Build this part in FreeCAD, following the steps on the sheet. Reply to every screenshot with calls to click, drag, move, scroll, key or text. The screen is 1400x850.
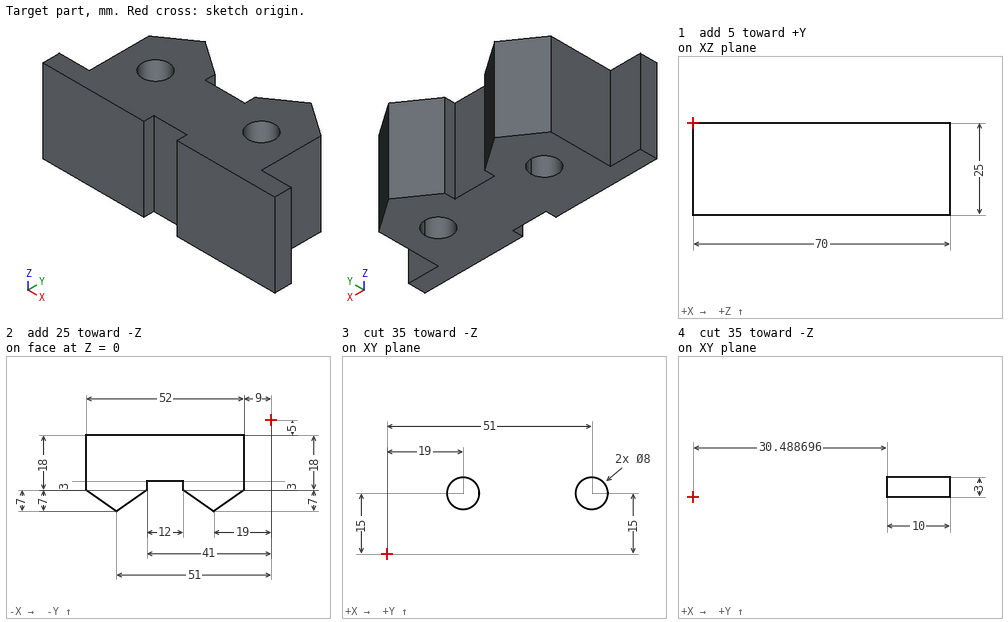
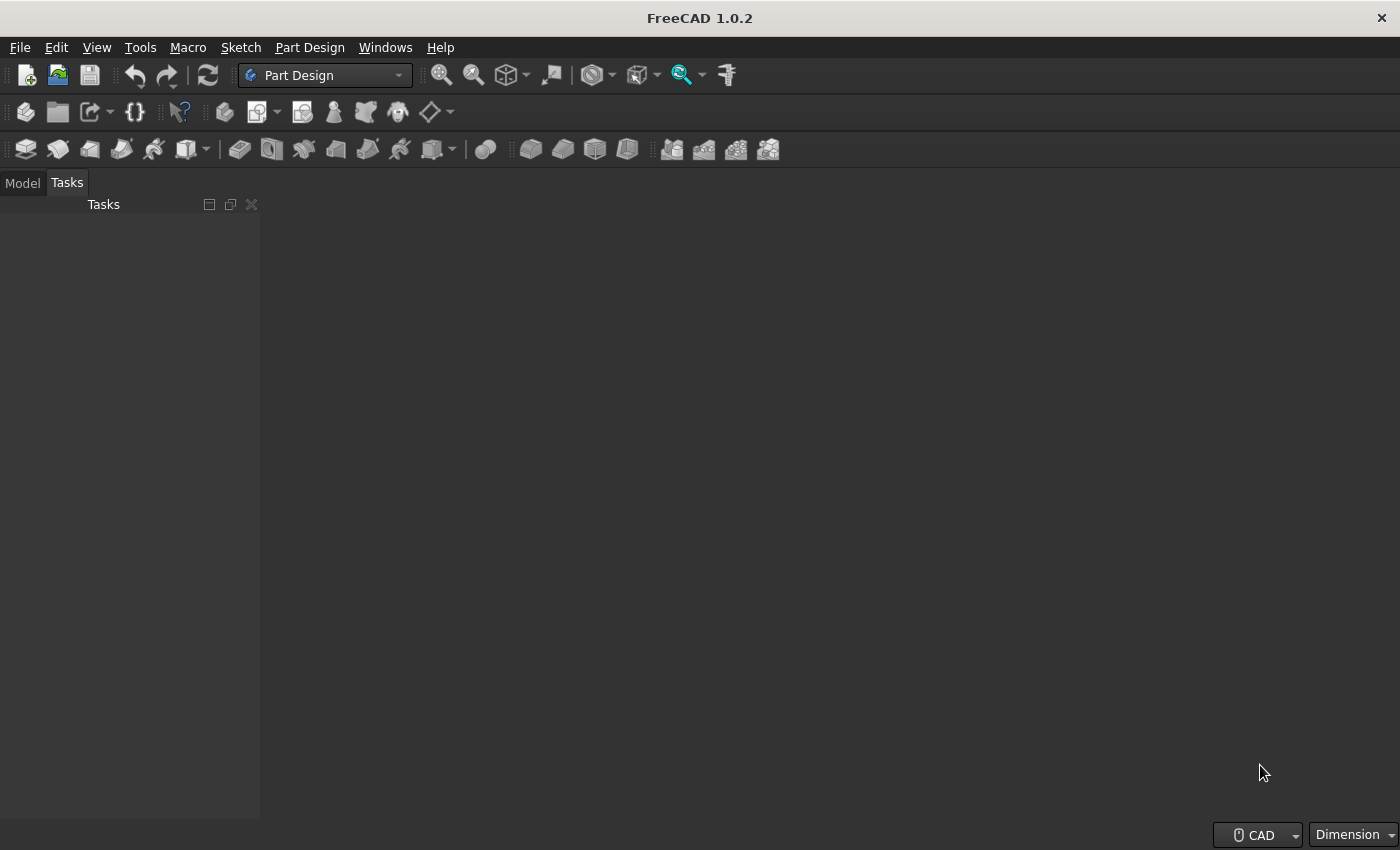
key(ctrl+n)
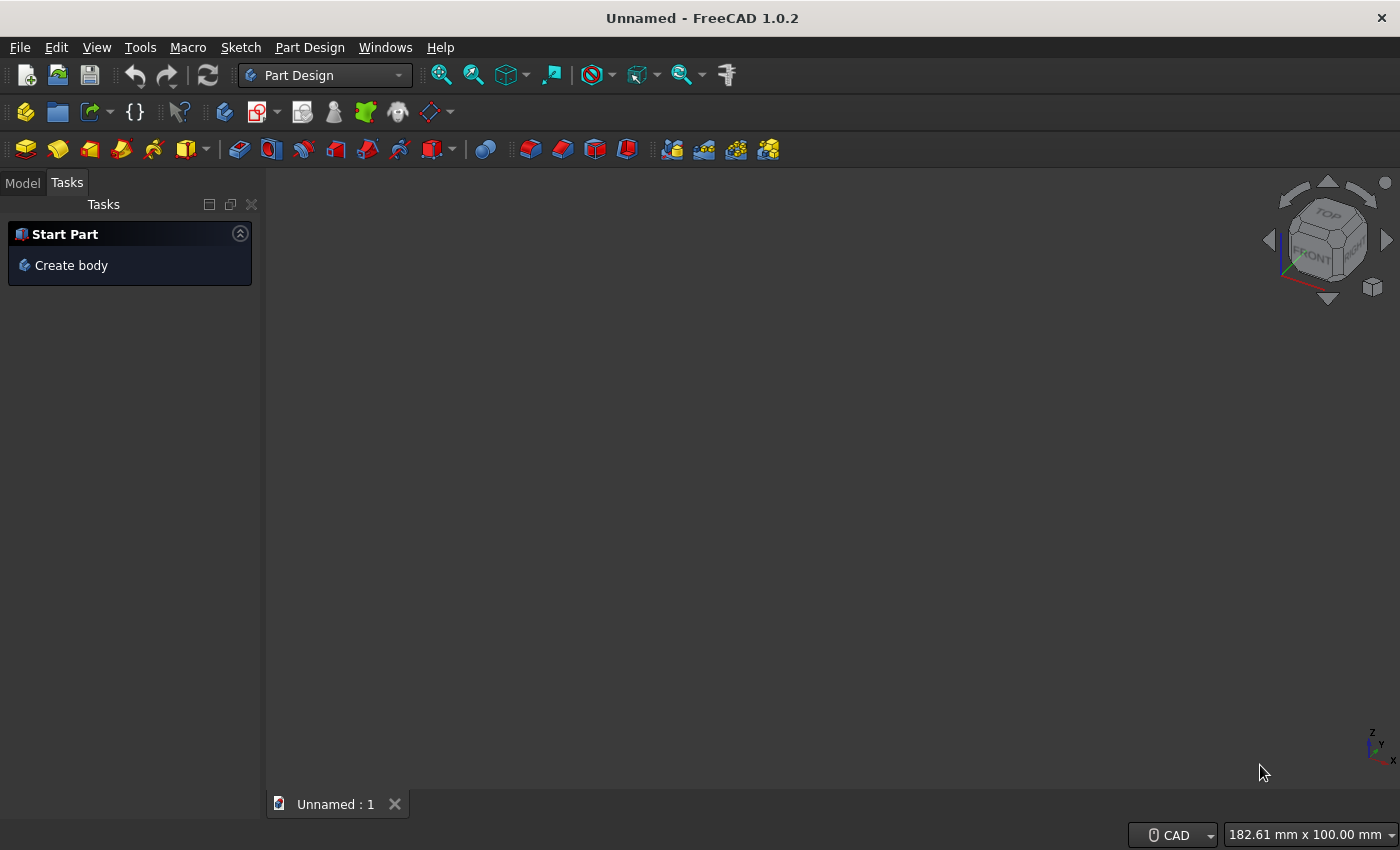
click(258, 112)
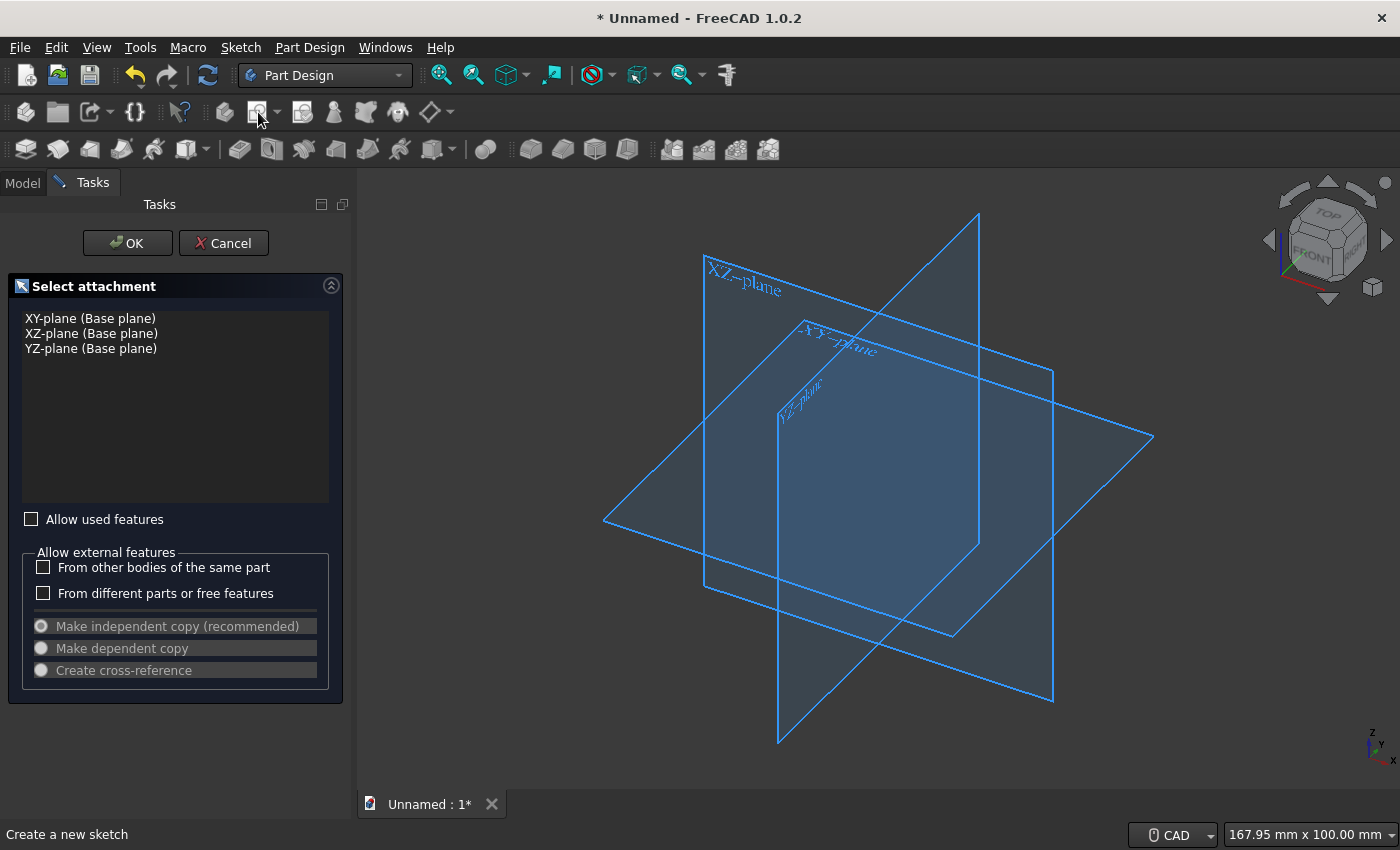
click(82, 334)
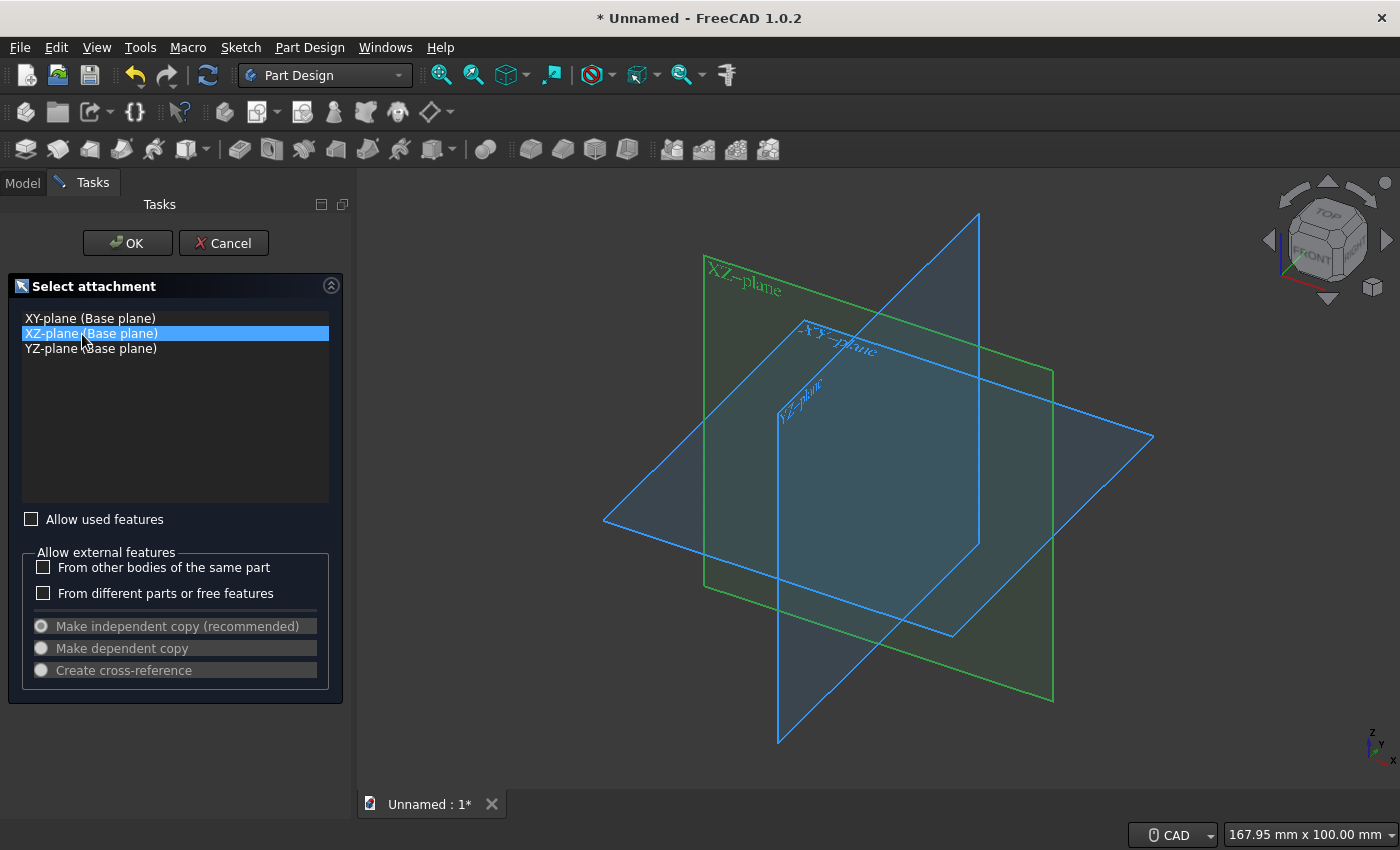
click(128, 243)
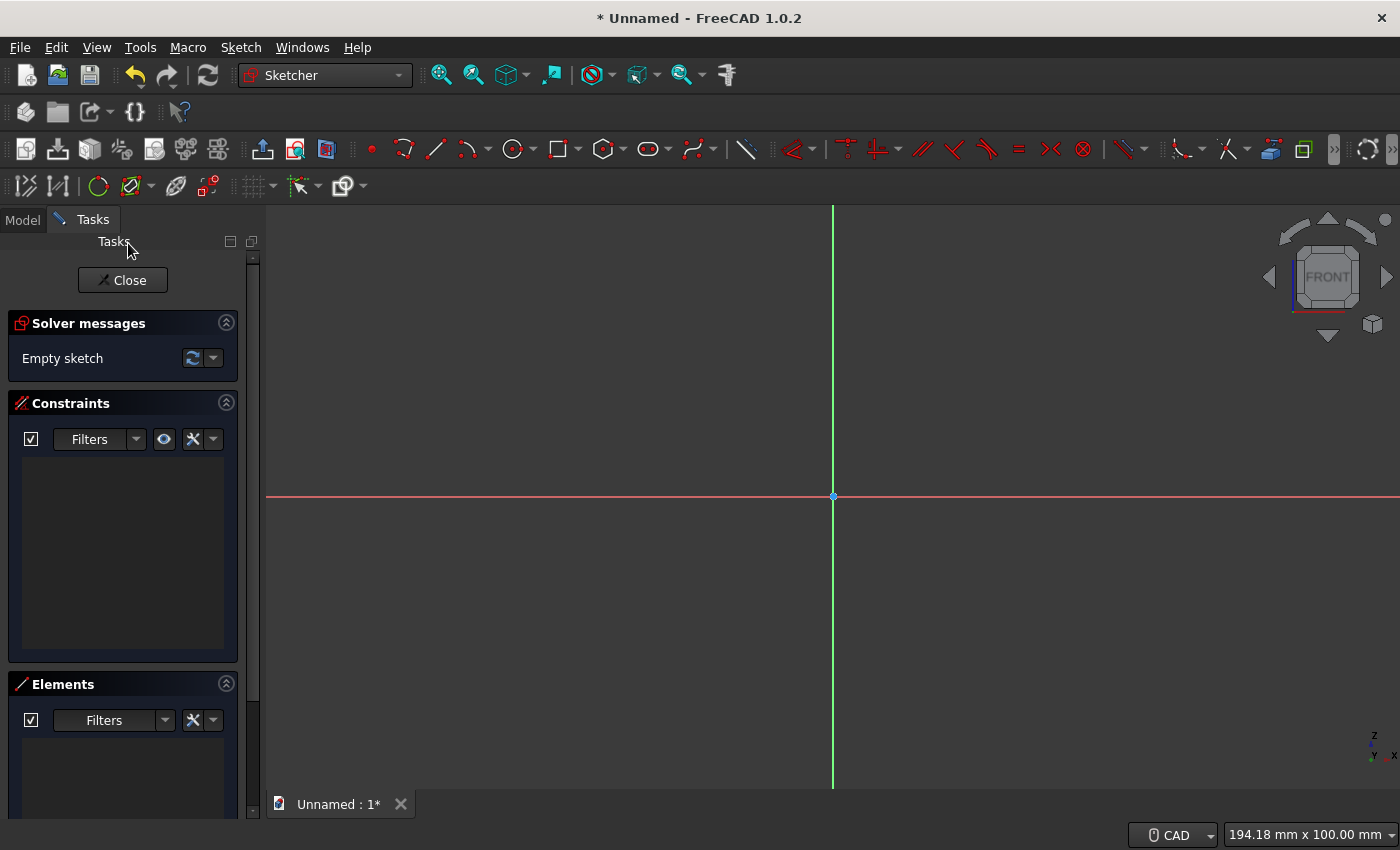
scroll(294, 233, down, 1)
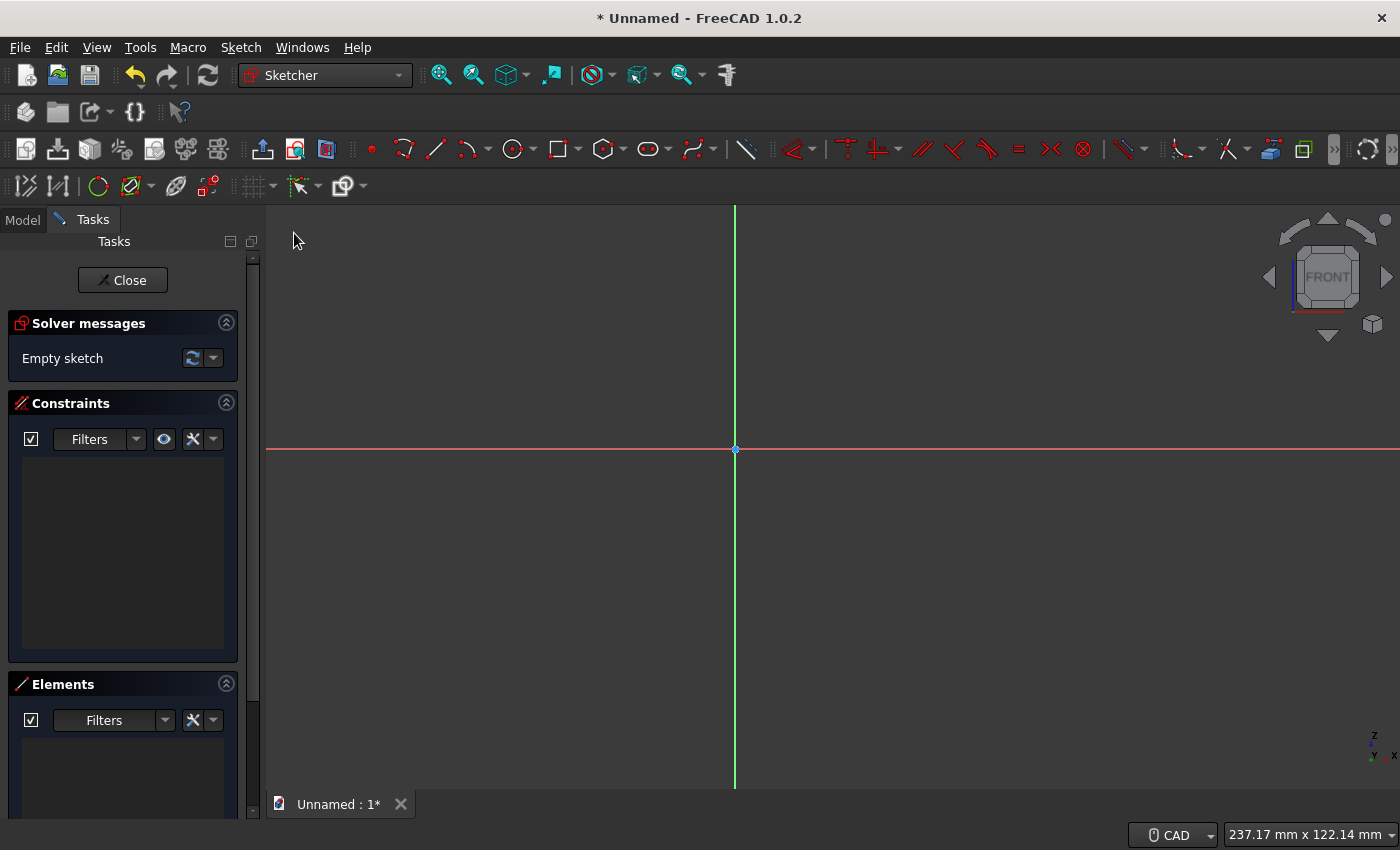
scroll(1071, 523, up, 3)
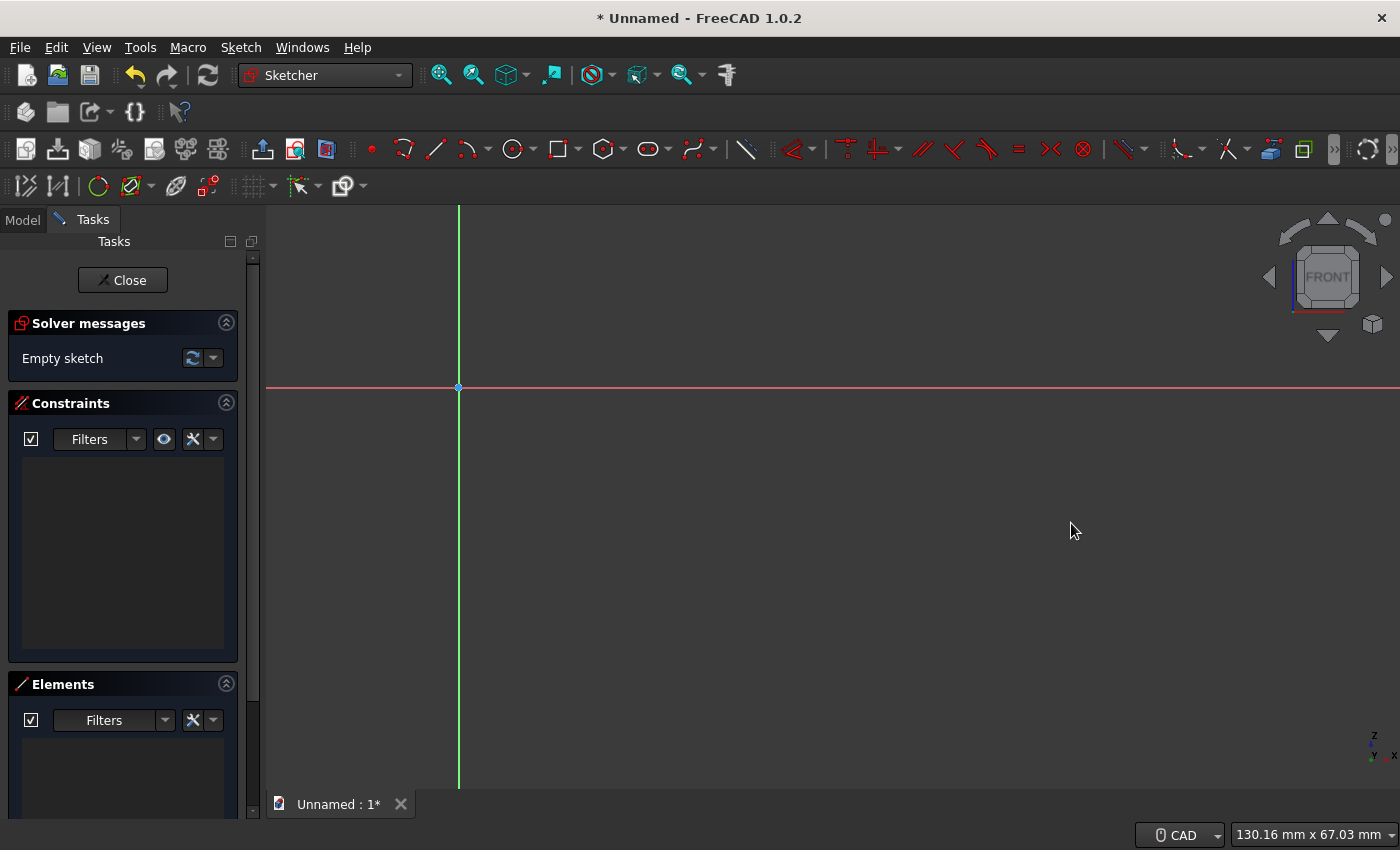
key(g)
key(r)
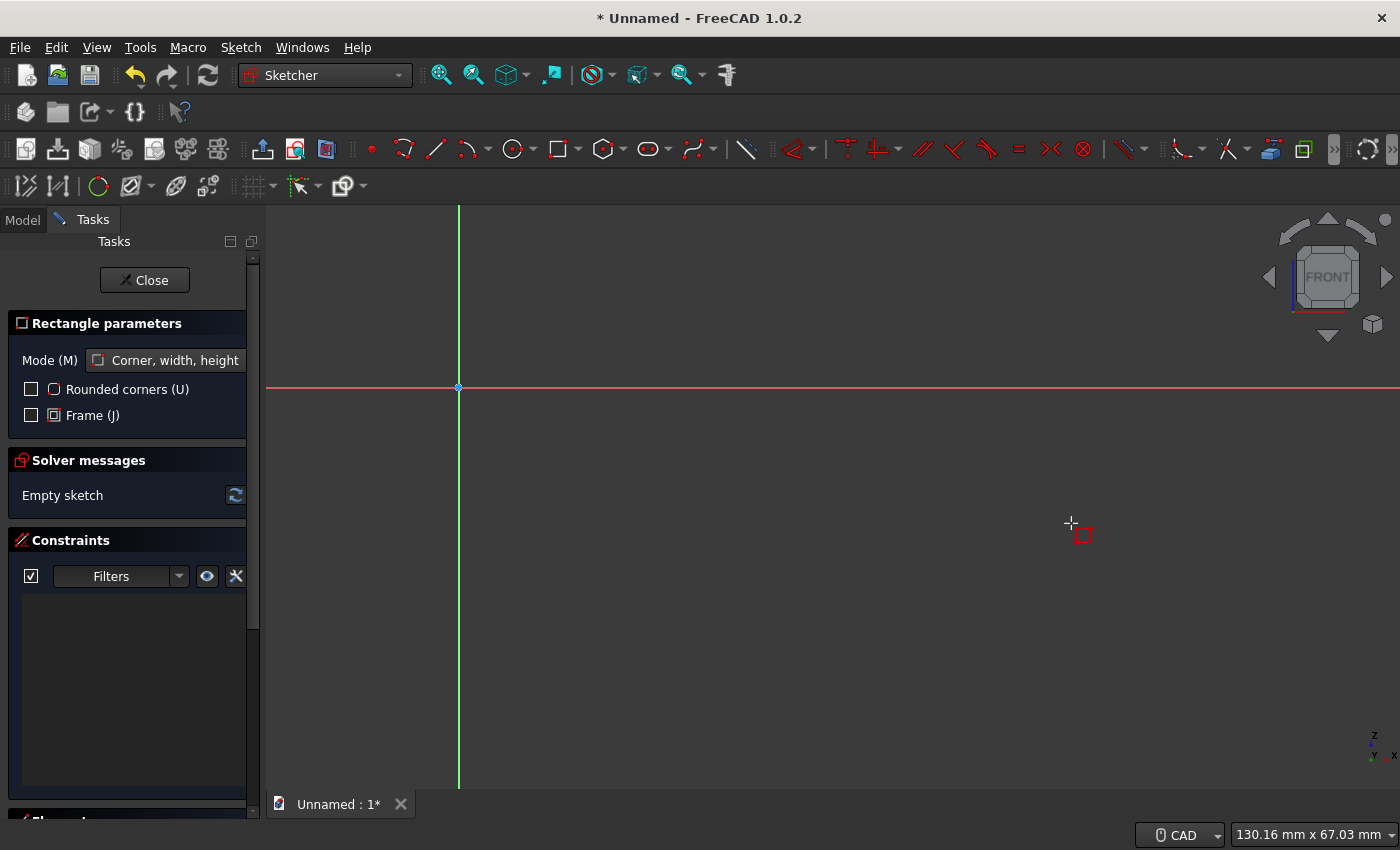
click(459, 388)
move(1069, 606)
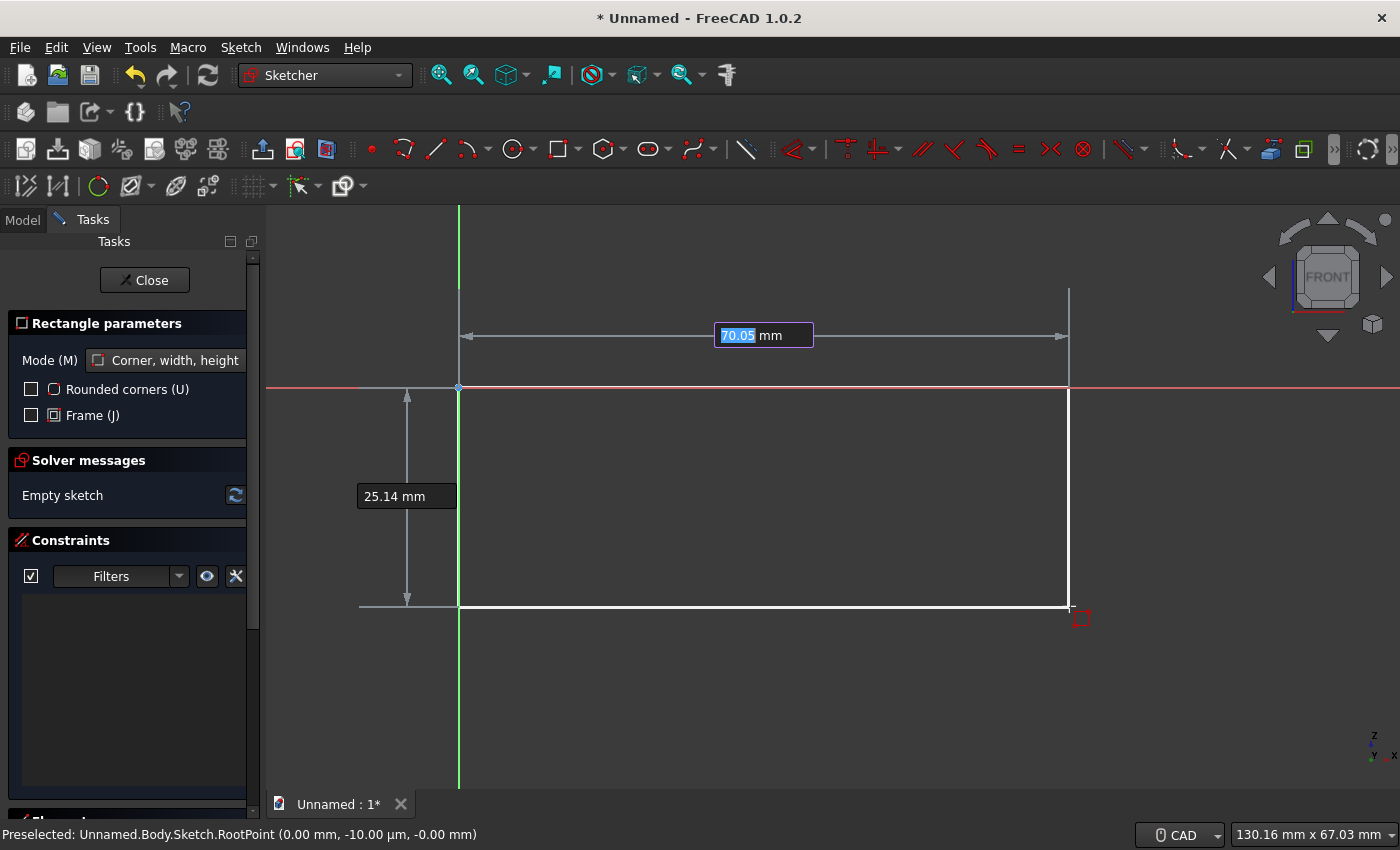
text(70)
key(Tab)
text(25)
key(Return)
key(Escape)